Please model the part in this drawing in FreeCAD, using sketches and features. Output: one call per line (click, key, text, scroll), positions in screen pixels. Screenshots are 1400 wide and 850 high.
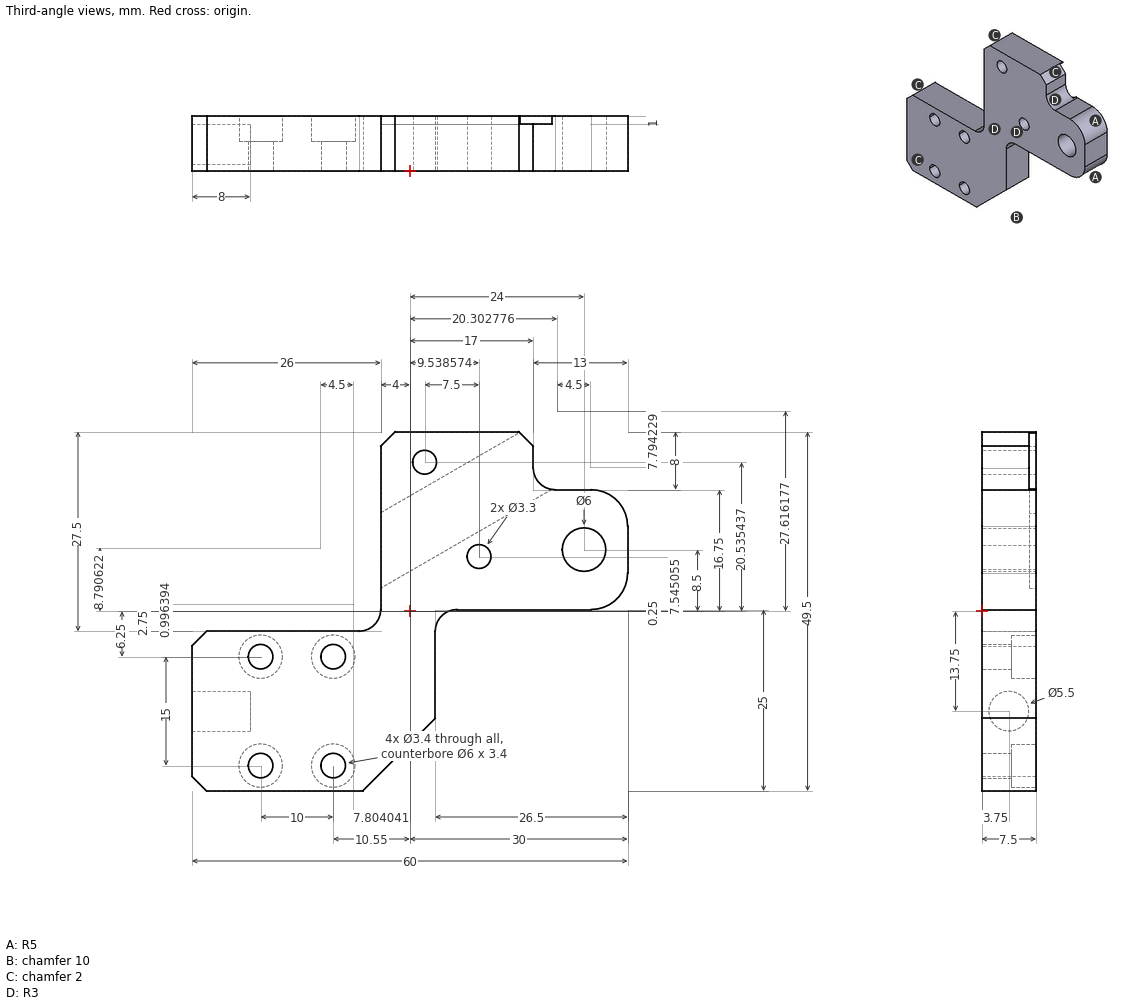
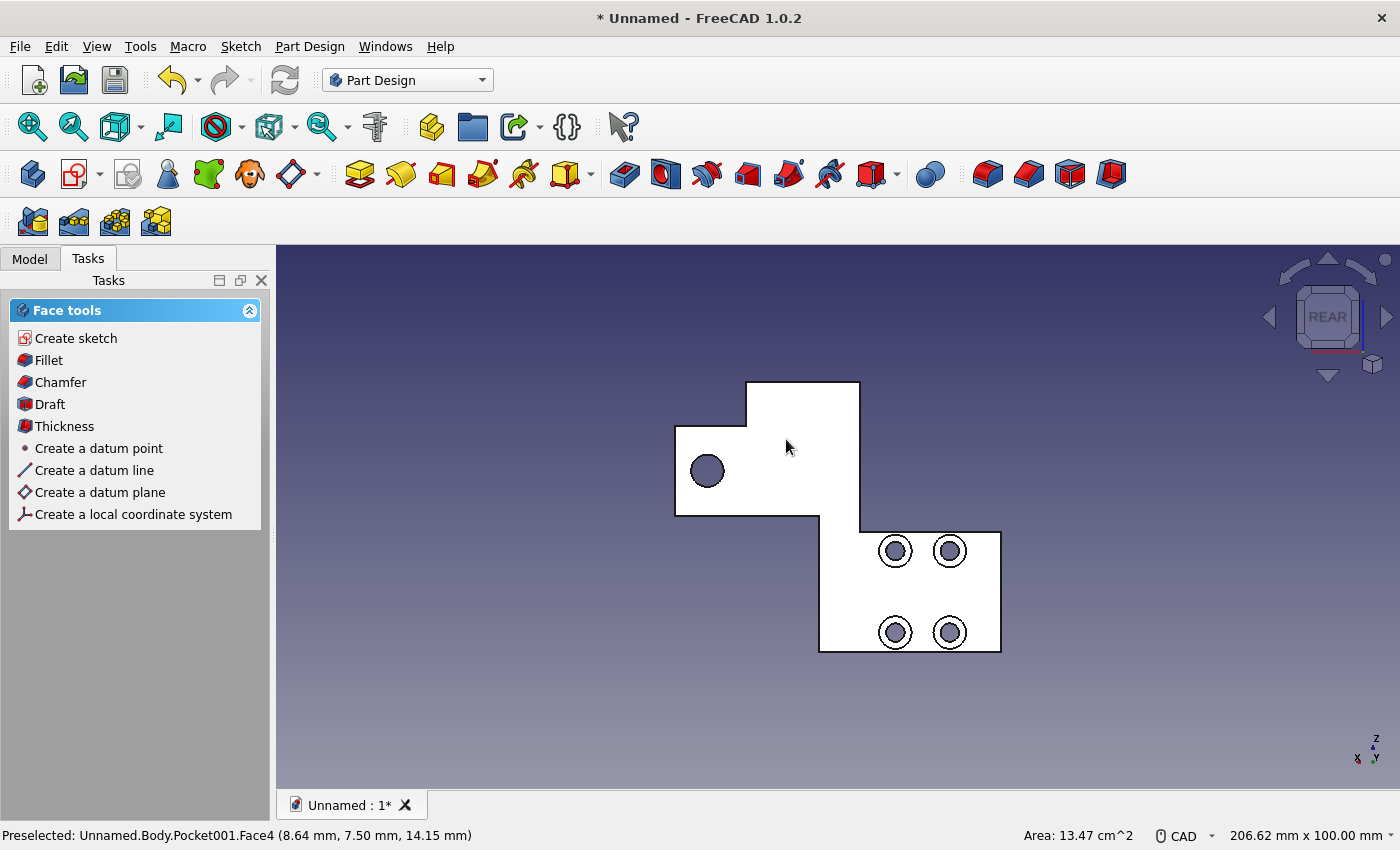
click(74, 174)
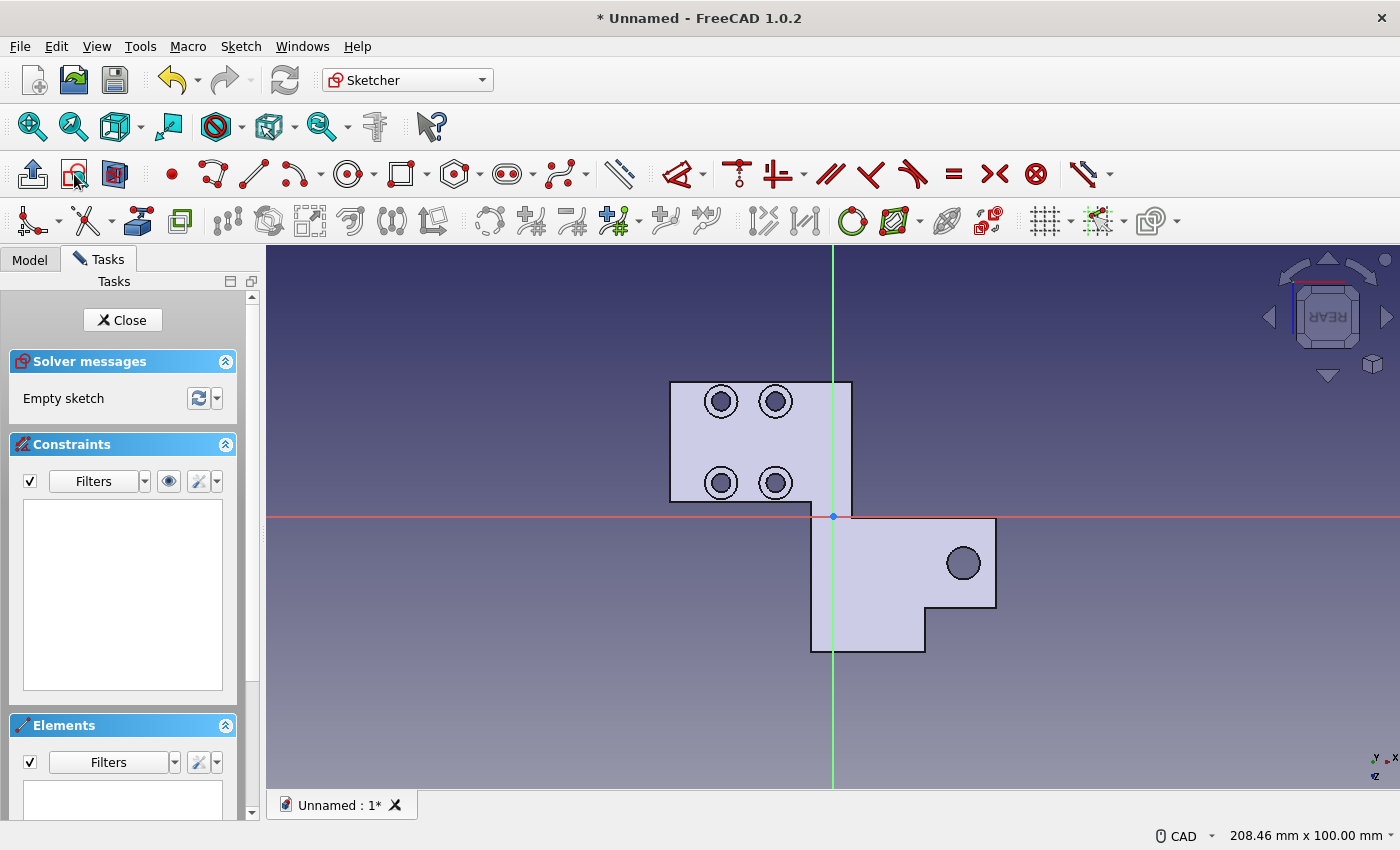
scroll(951, 653, up, 4)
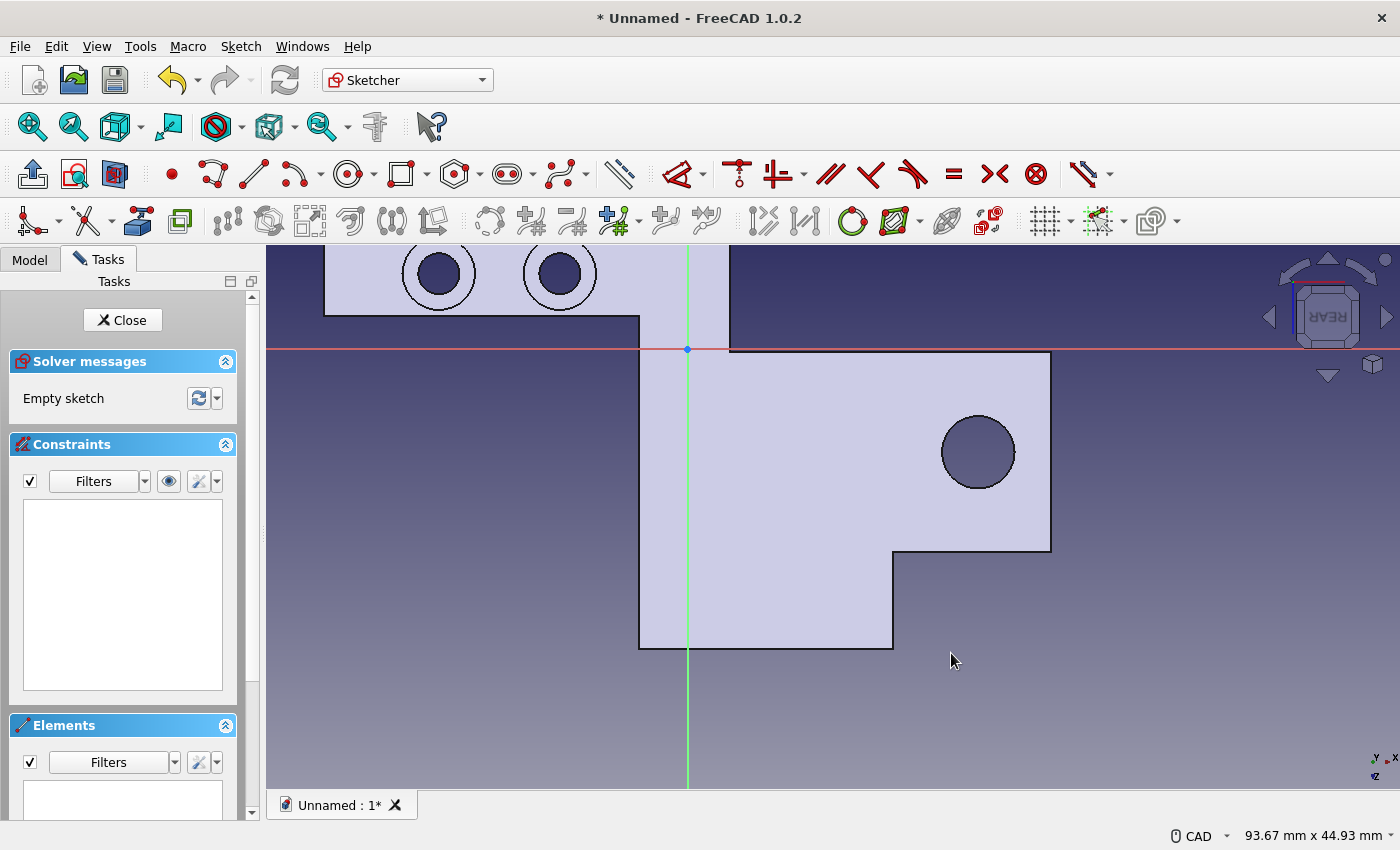
click(213, 174)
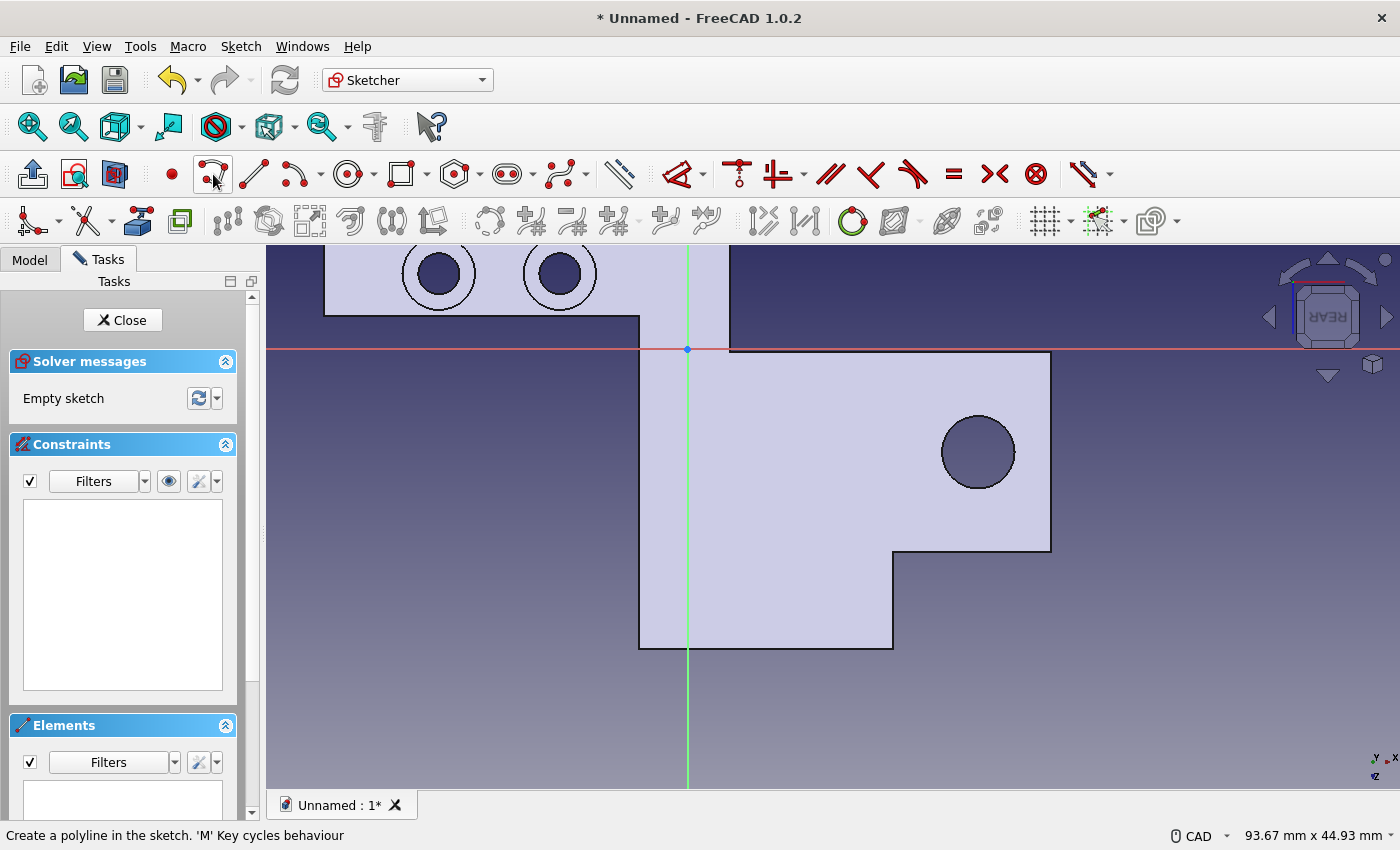
scroll(593, 361, up, 2)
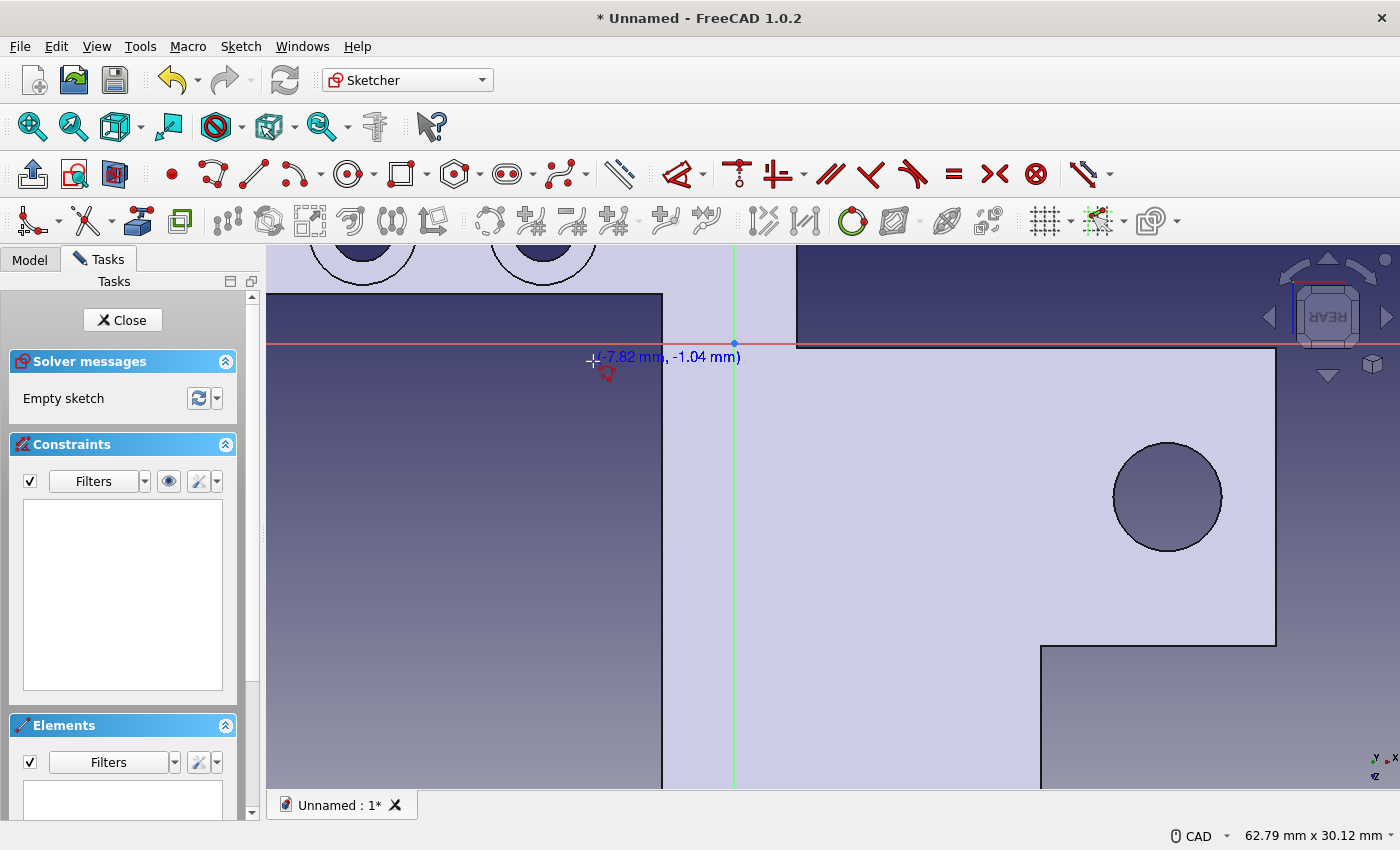
click(593, 362)
click(512, 502)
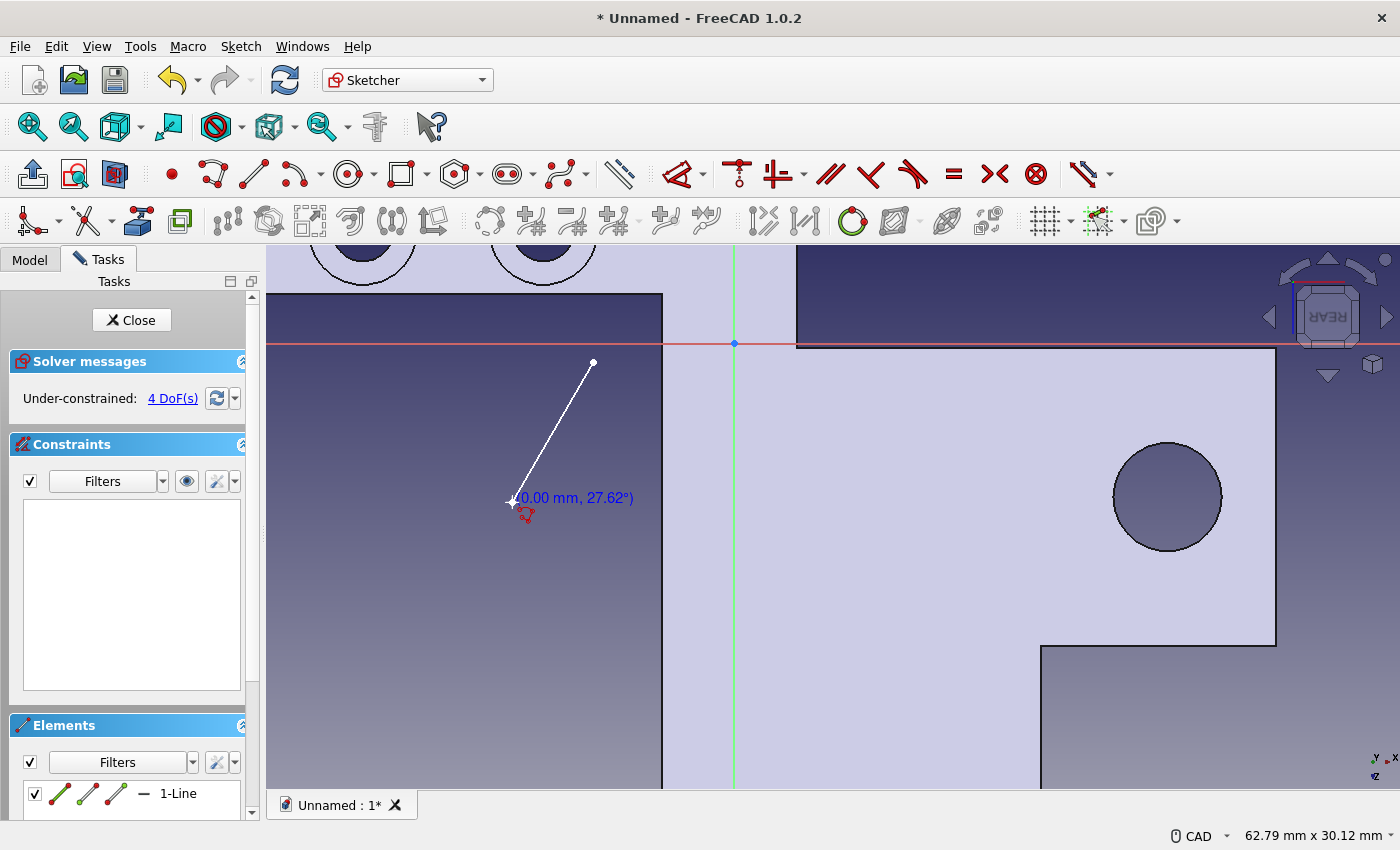
scroll(597, 362, down, 2)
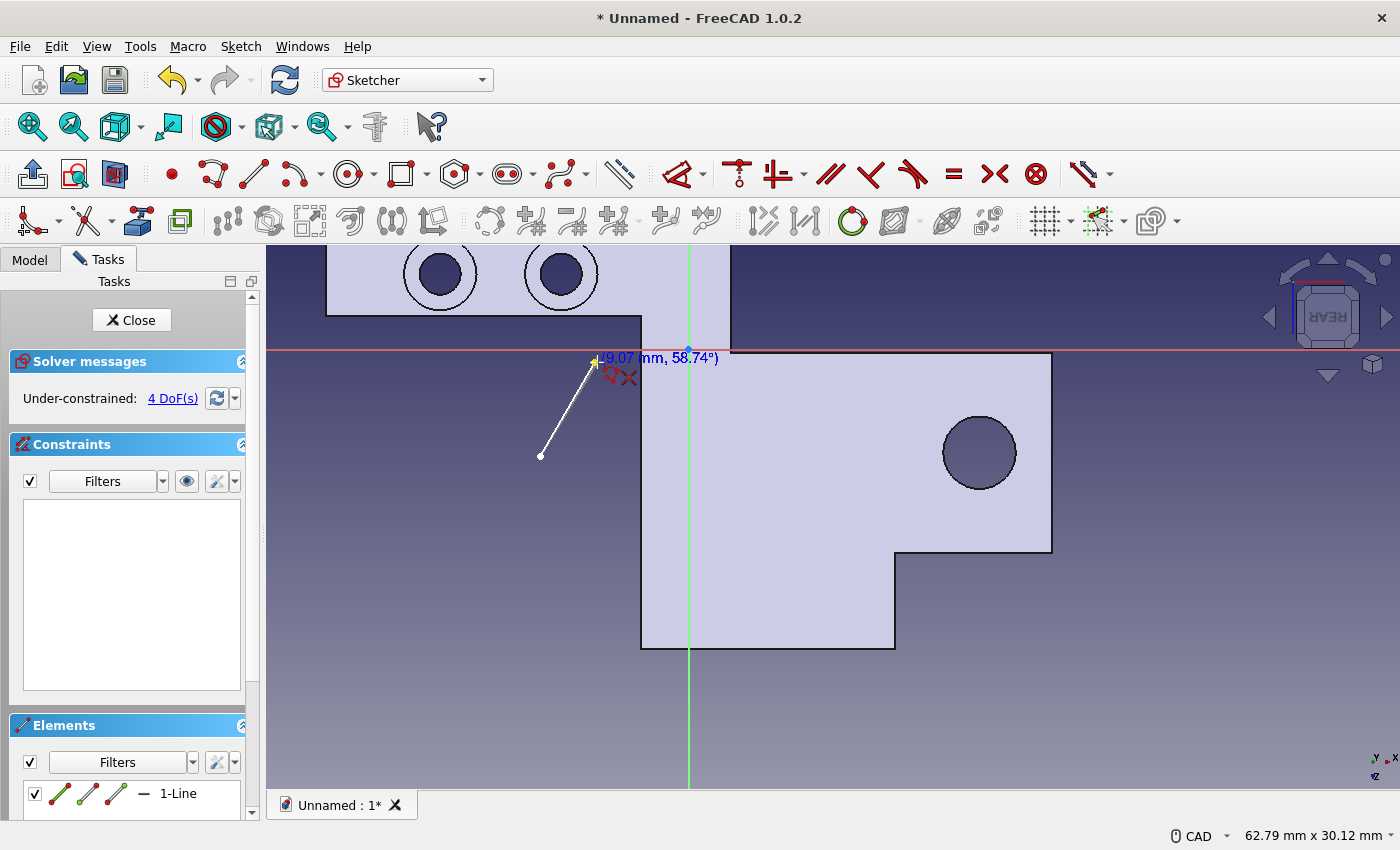
click(935, 684)
click(989, 590)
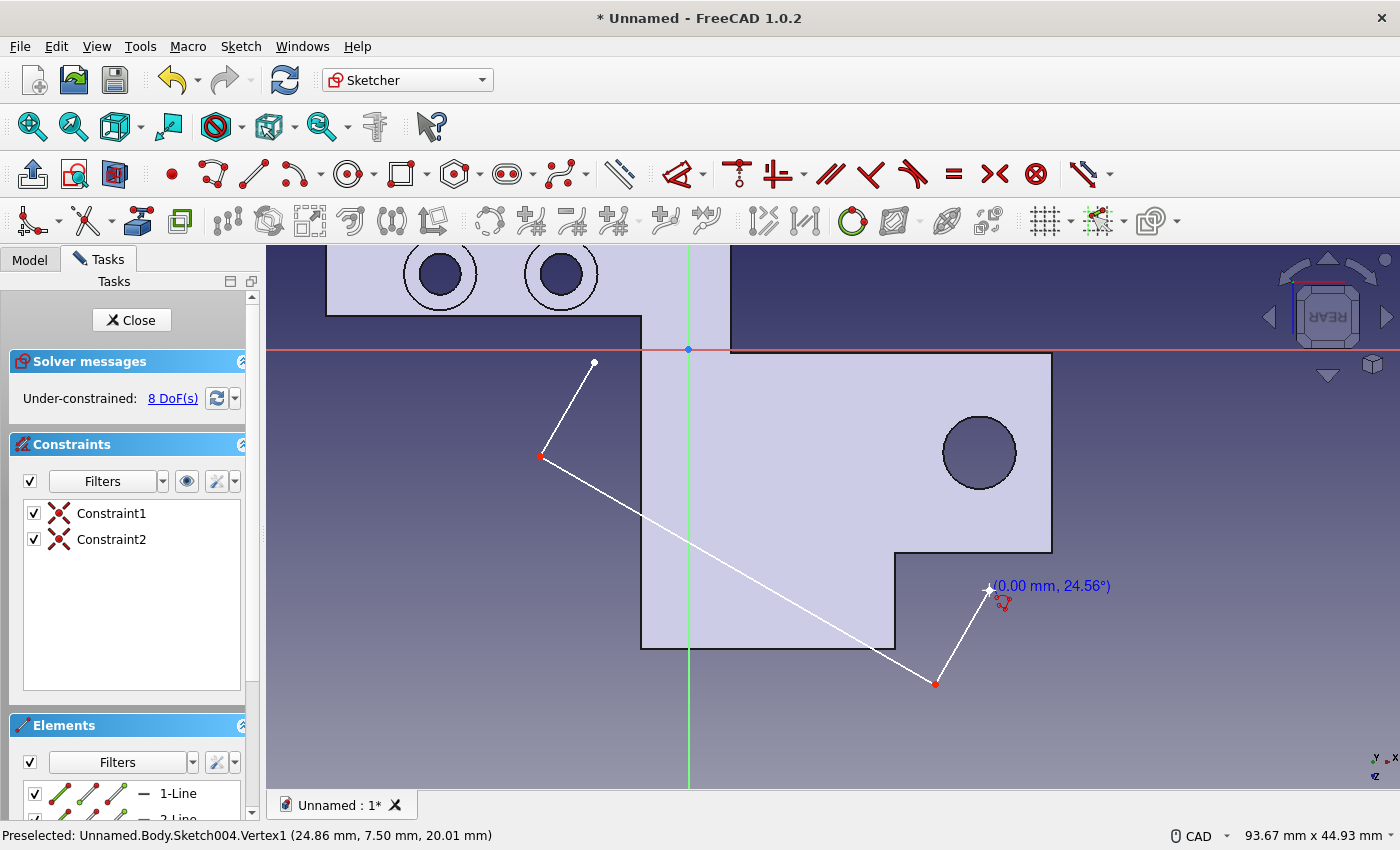
scroll(594, 362, up, 2)